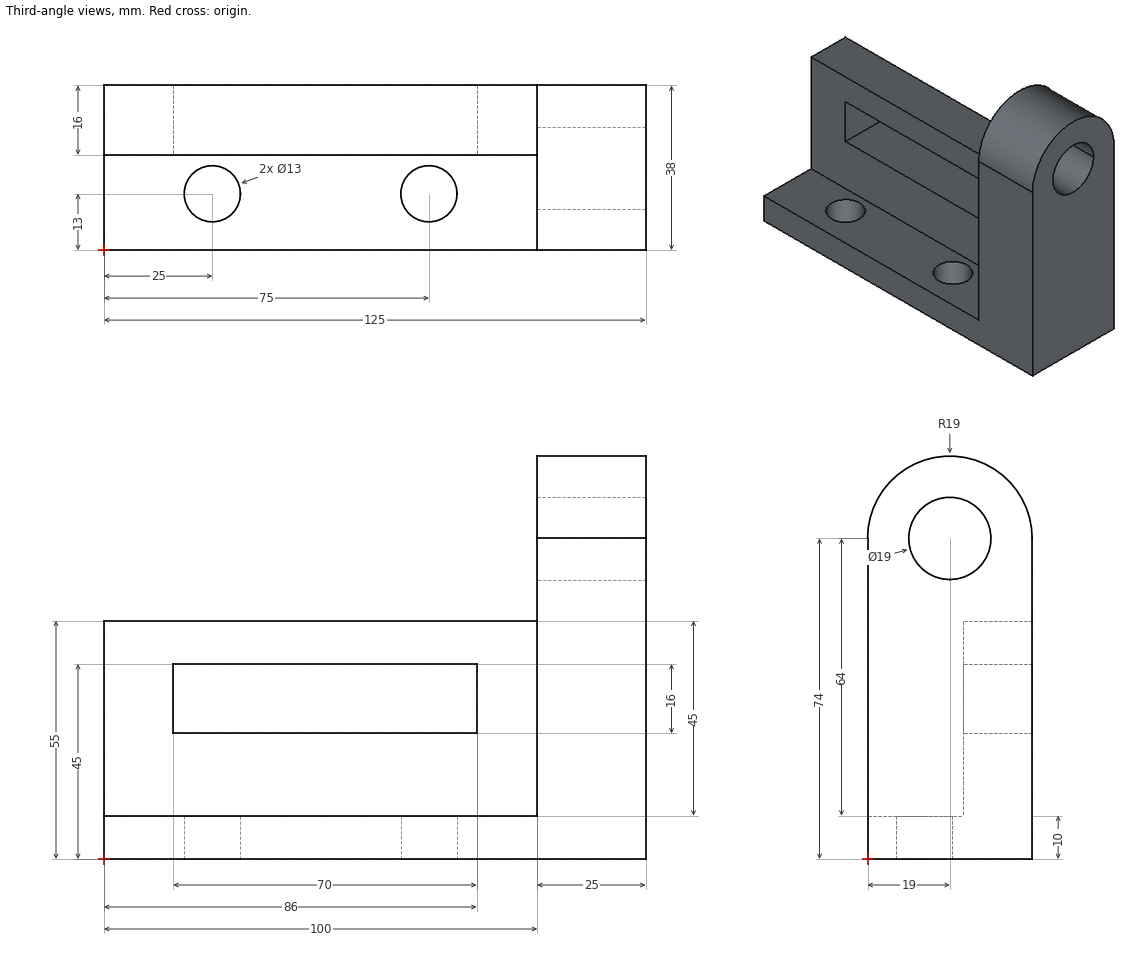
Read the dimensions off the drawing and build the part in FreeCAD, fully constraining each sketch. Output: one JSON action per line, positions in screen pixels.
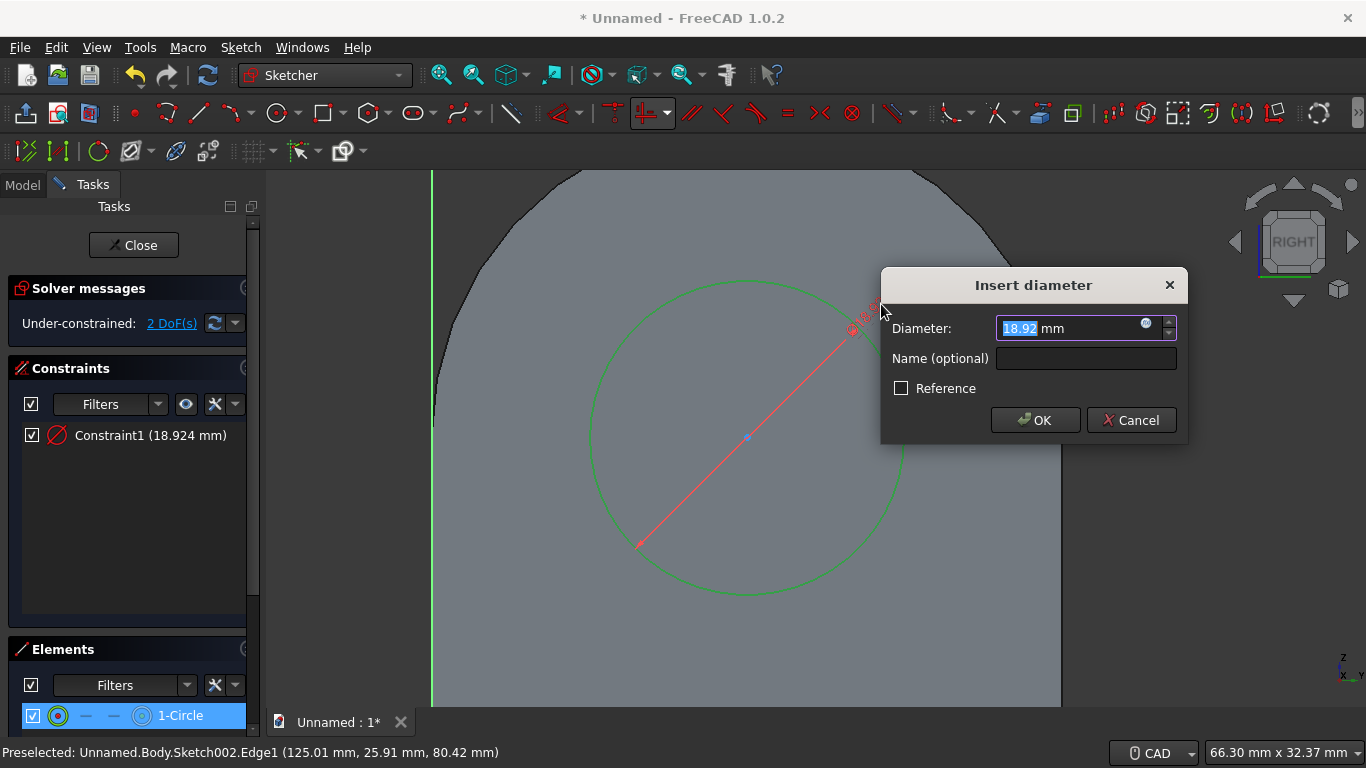
{"action": "type", "text": "19"}
{"action": "key", "text": "Return"}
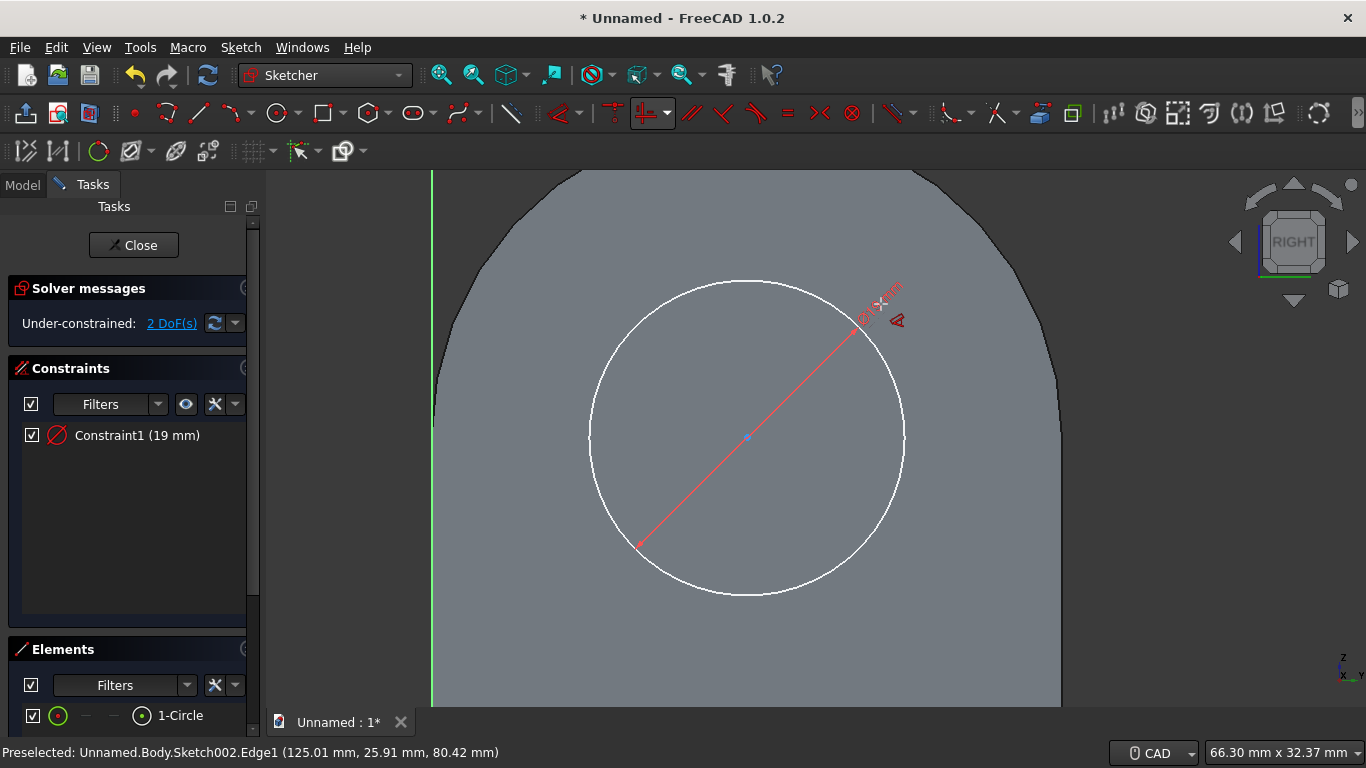
{"action": "left_click", "coordinate": [747, 438]}
{"action": "left_click", "coordinate": [517, 404]}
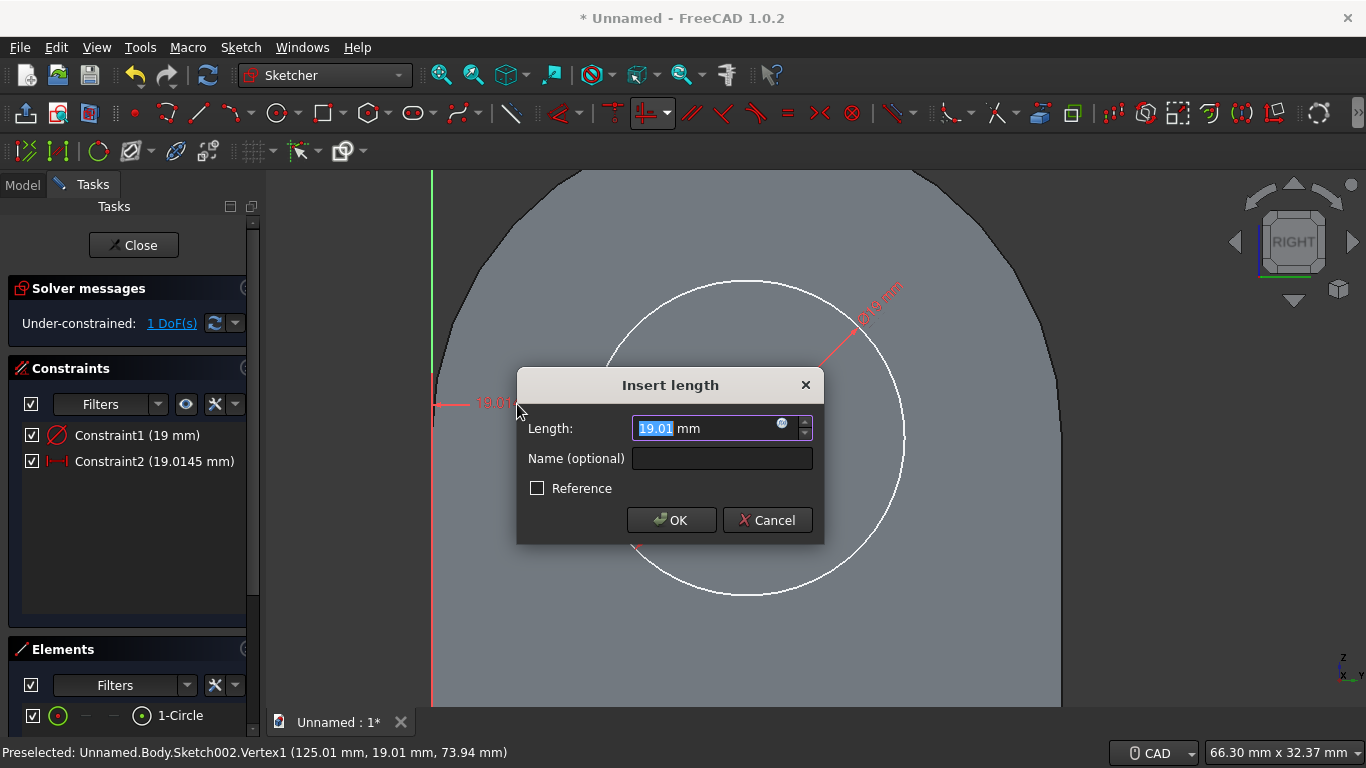
{"action": "type", "text": "19"}
{"action": "key", "text": "Return"}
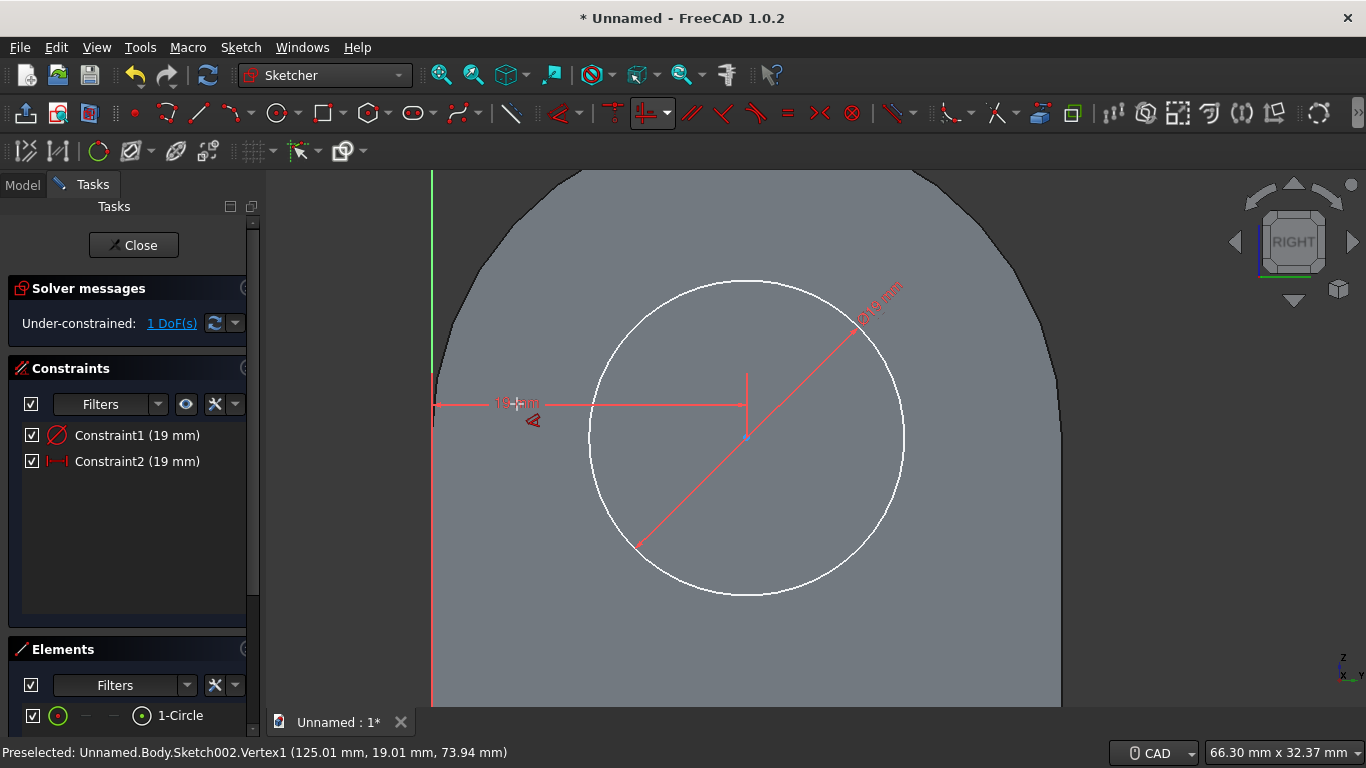
{"action": "left_click", "coordinate": [747, 438]}
{"action": "left_click", "coordinate": [398, 559]}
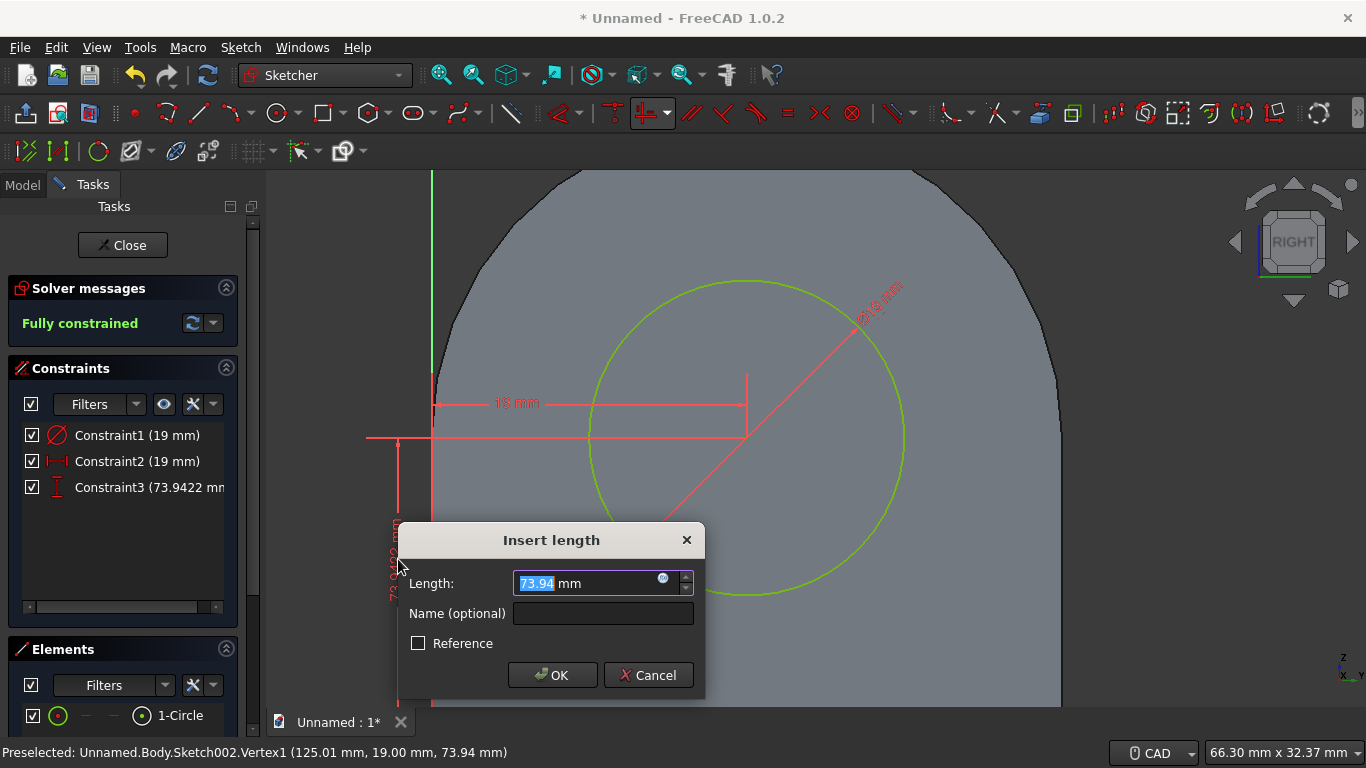
{"action": "type", "text": "74"}
{"action": "key", "text": "Return"}
{"action": "key", "text": "Escape"}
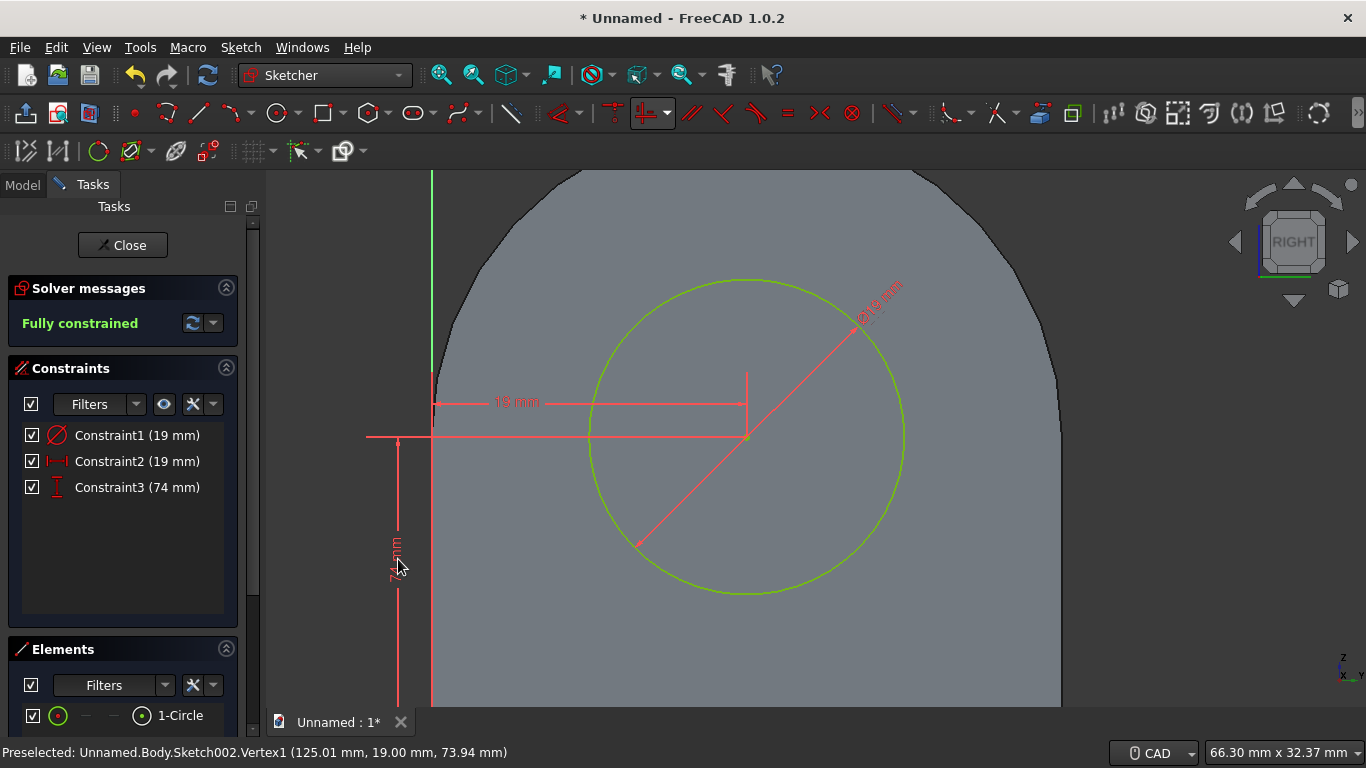
{"action": "left_click", "coordinate": [123, 245]}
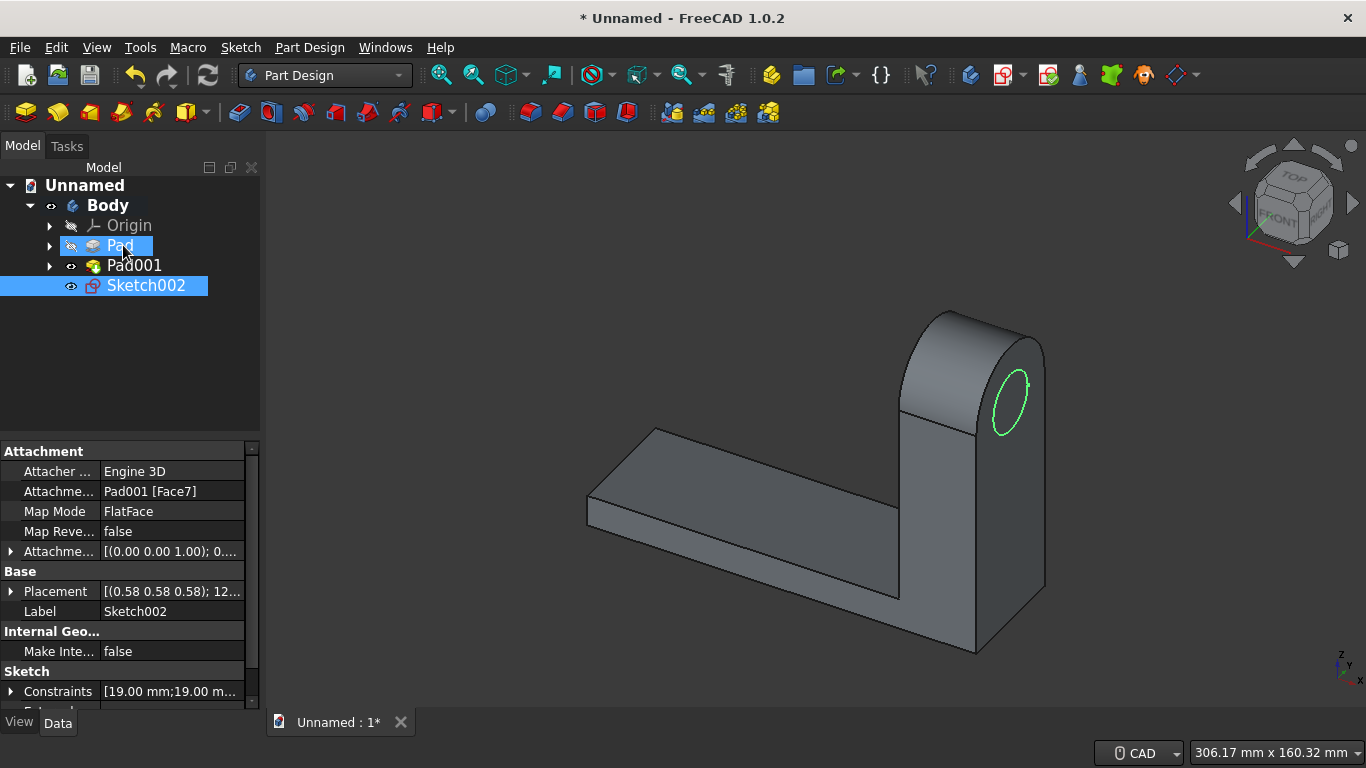
{"action": "left_click", "coordinate": [240, 112]}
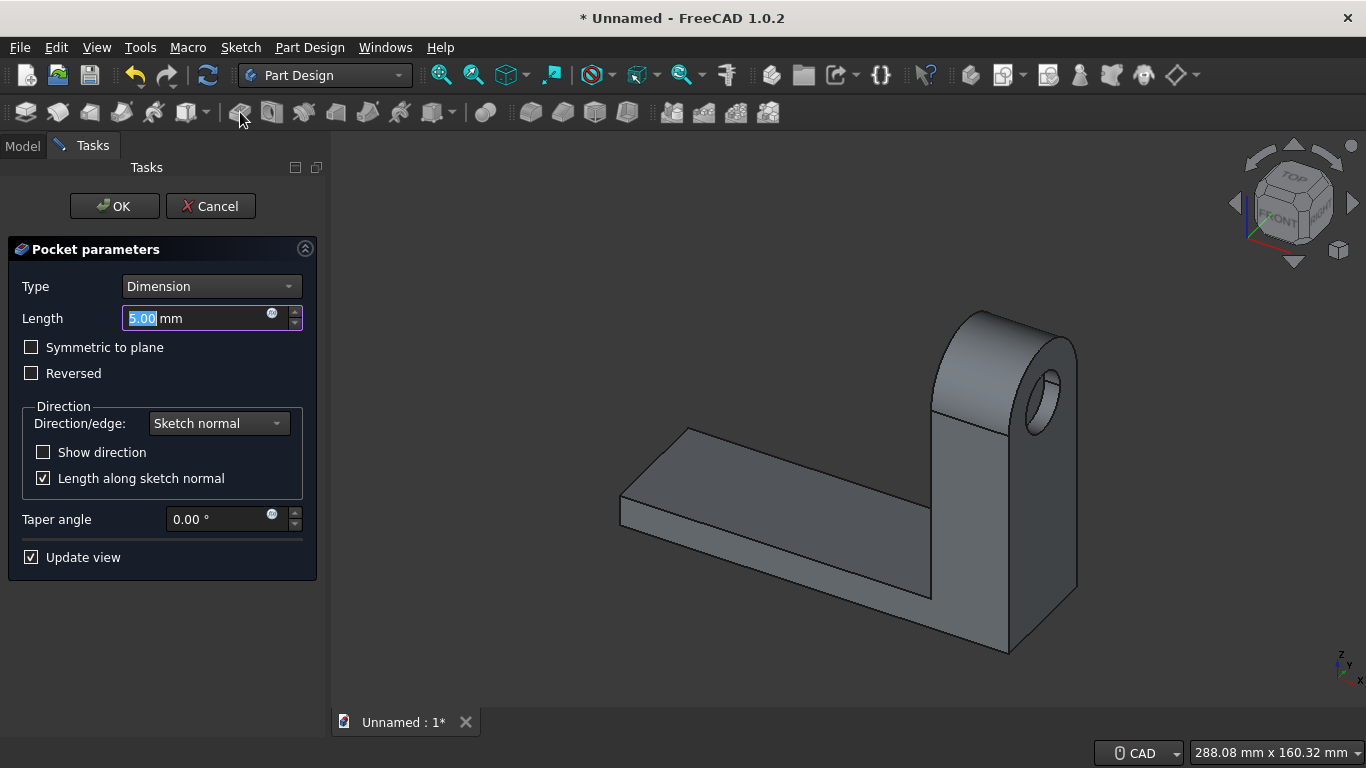
{"action": "type", "text": "25"}
{"action": "key", "text": "Tab"}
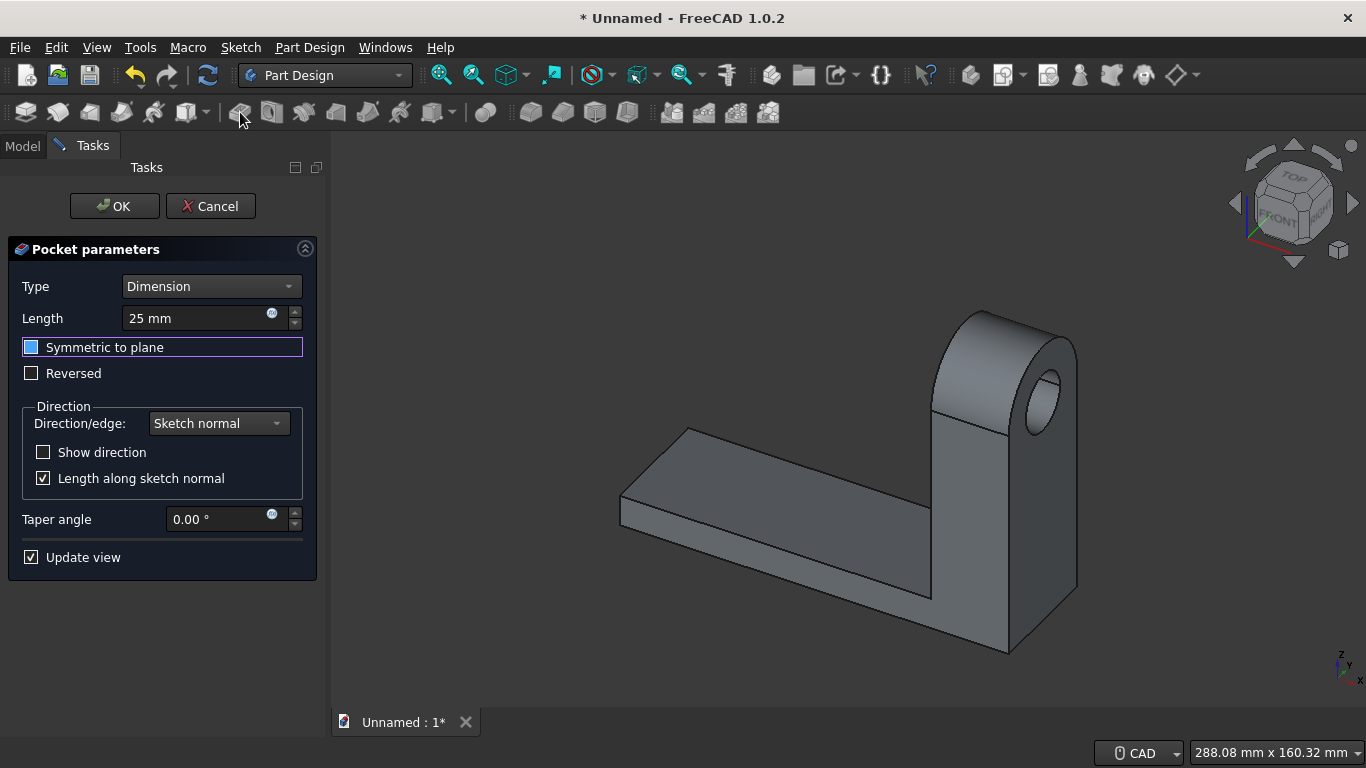
{"action": "left_click", "coordinate": [115, 206]}